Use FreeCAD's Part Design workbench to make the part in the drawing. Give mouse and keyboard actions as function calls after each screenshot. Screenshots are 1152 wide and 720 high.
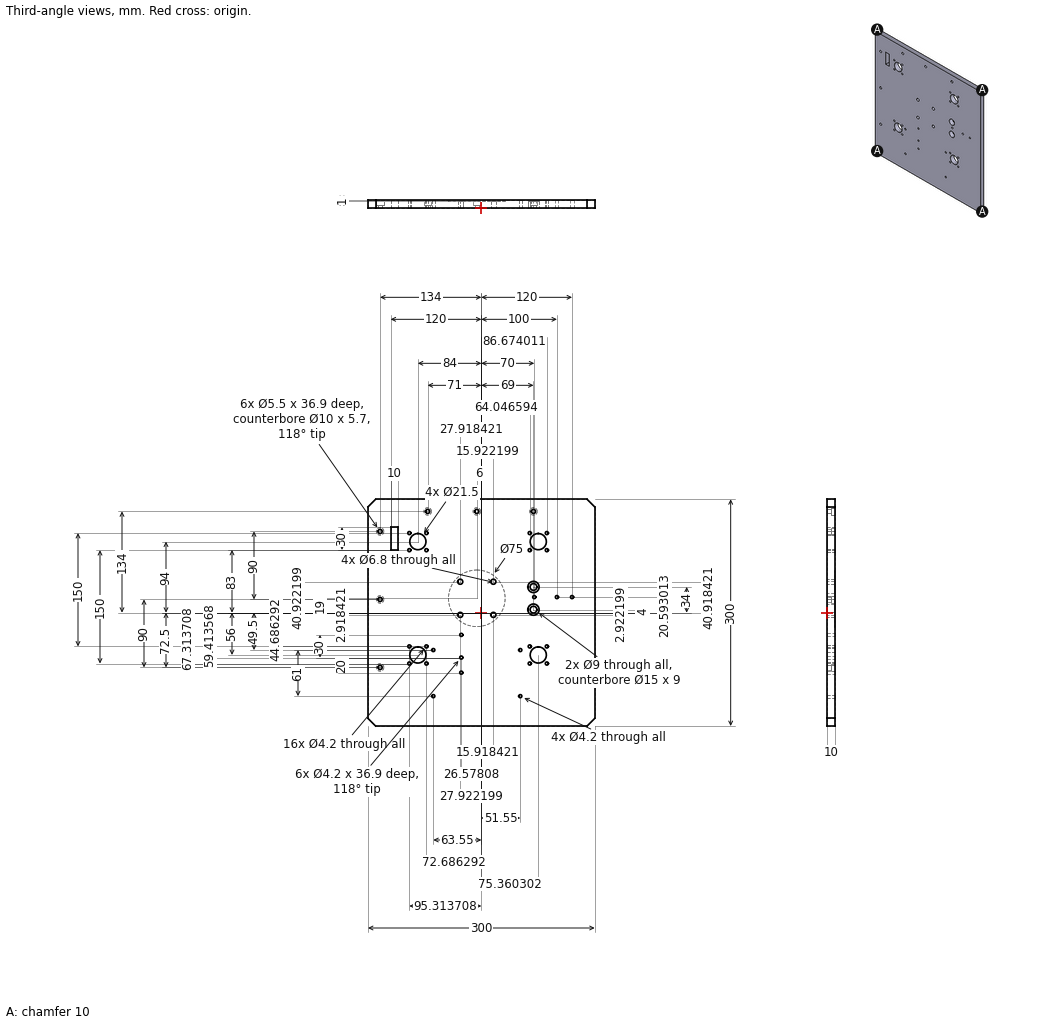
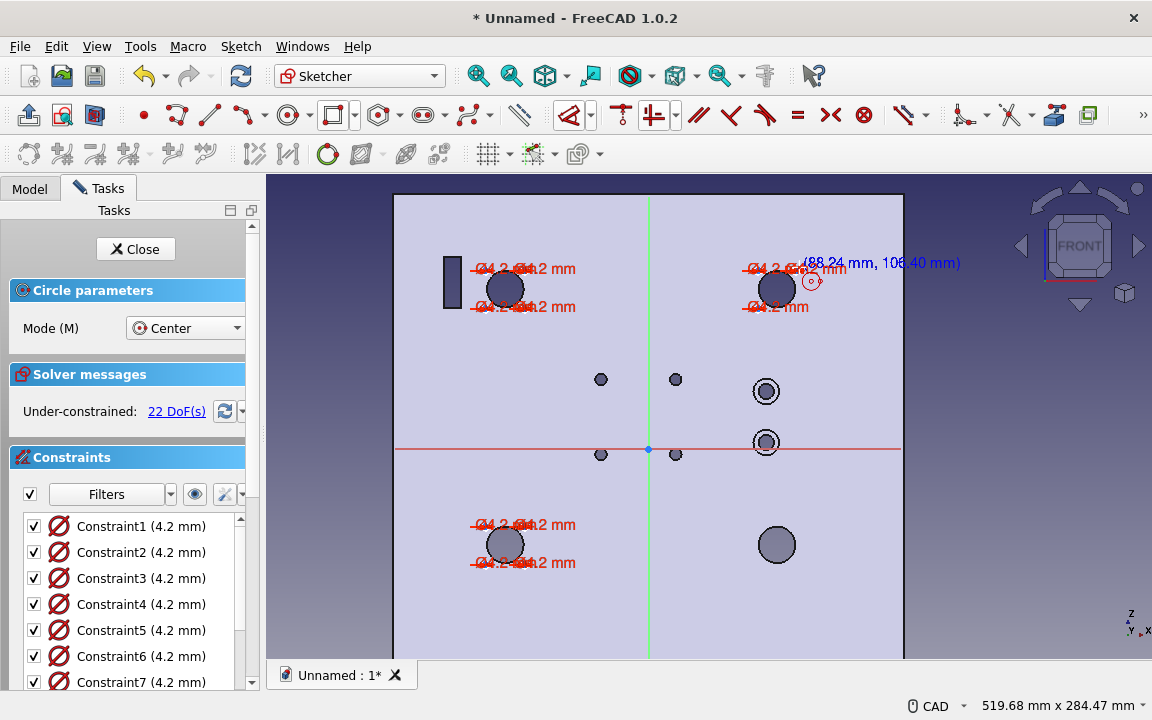
scroll(796, 308, up, 10)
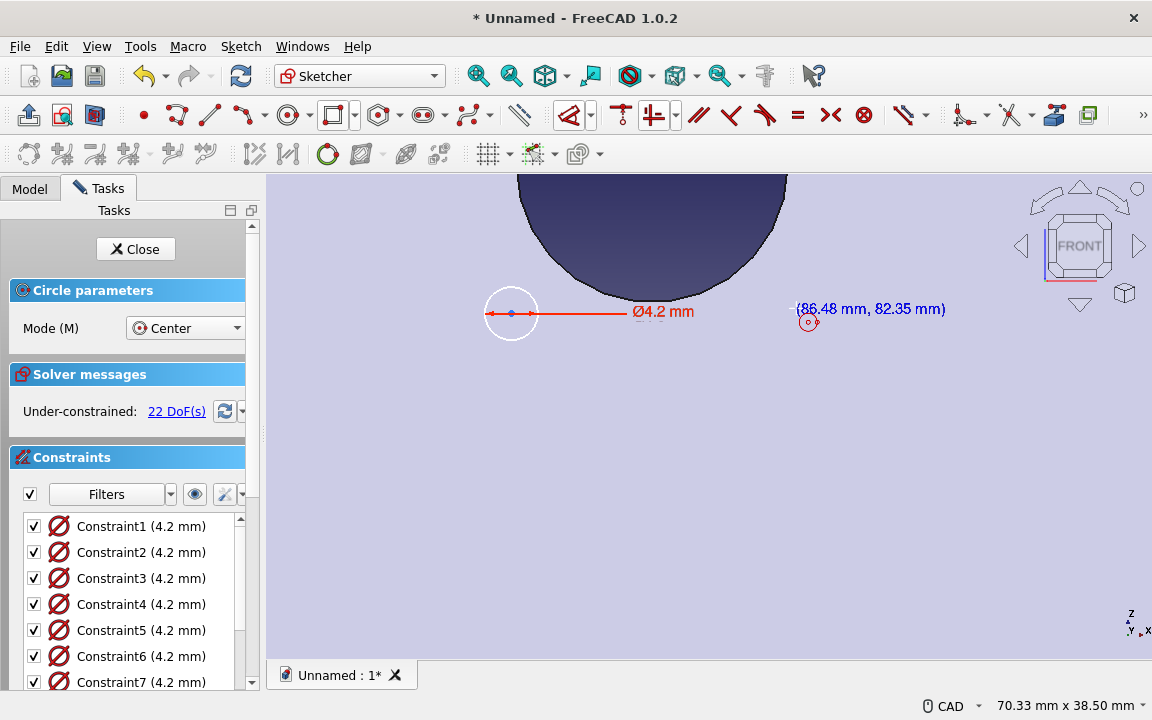
scroll(796, 308, down, 10)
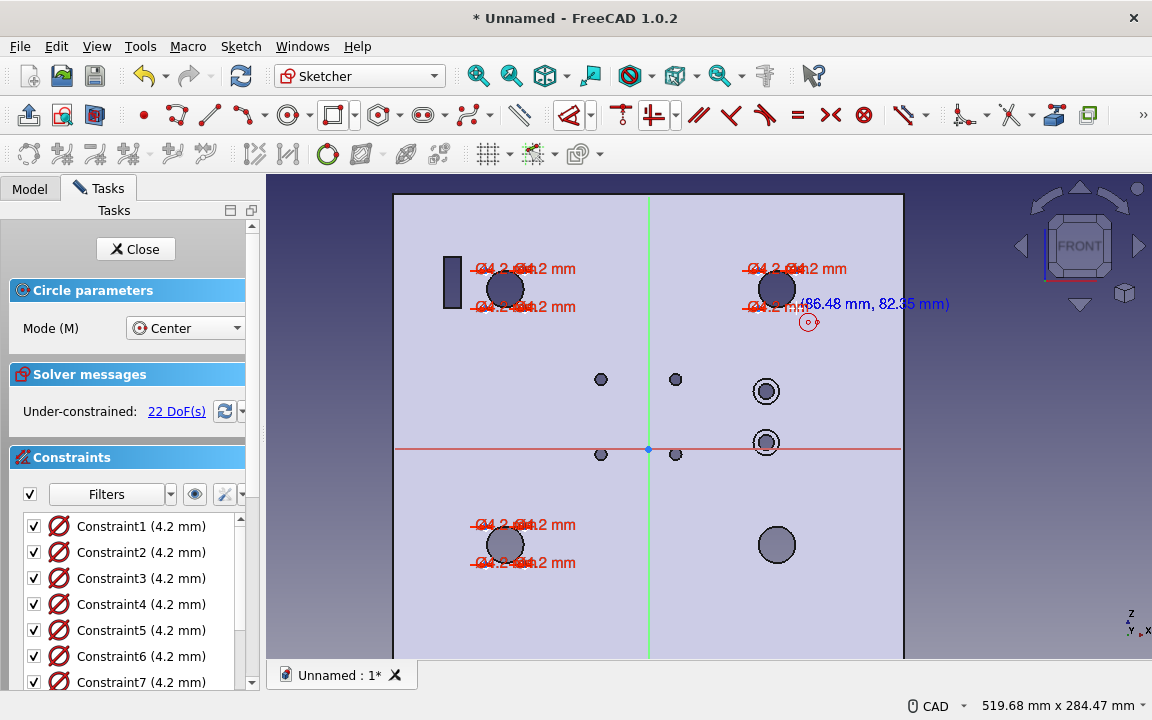
click(796, 308)
move(799, 306)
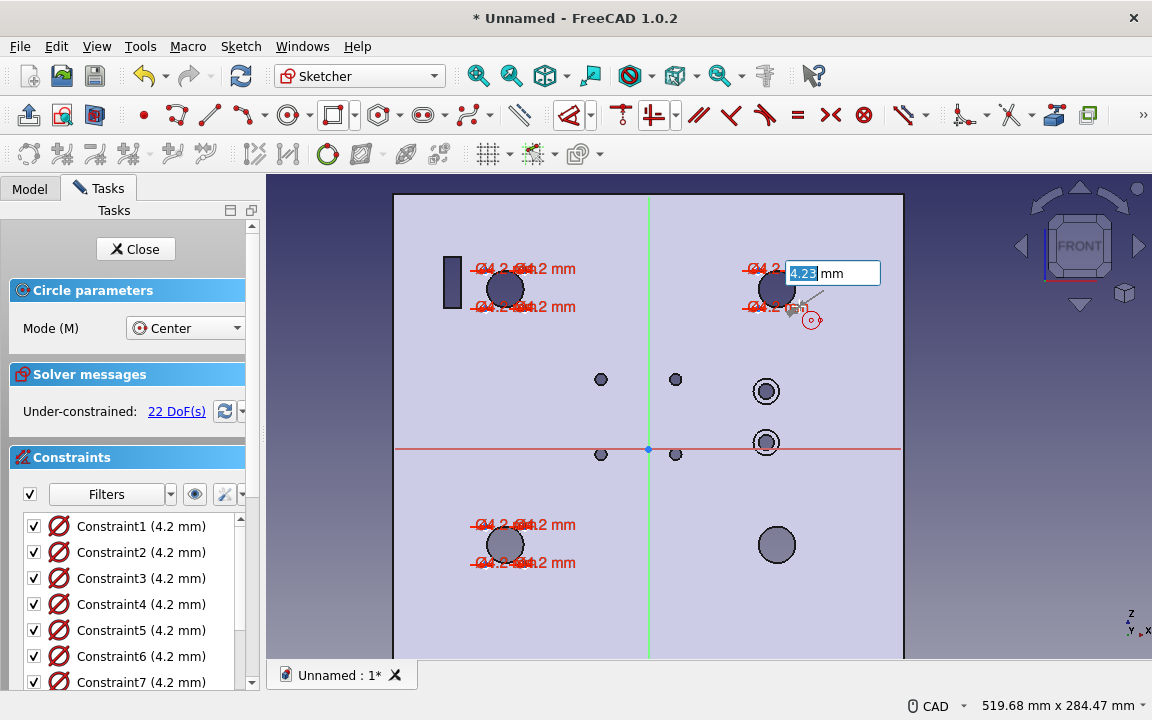
text(4.2)
key(Return)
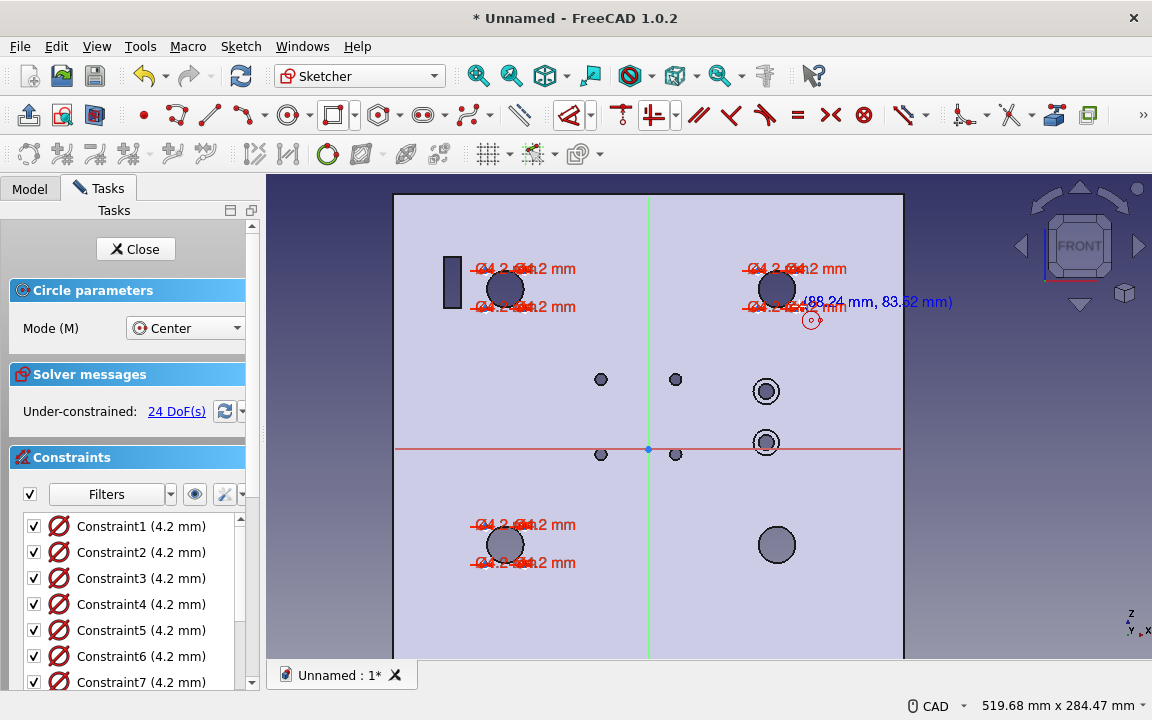
scroll(758, 564, up, 10)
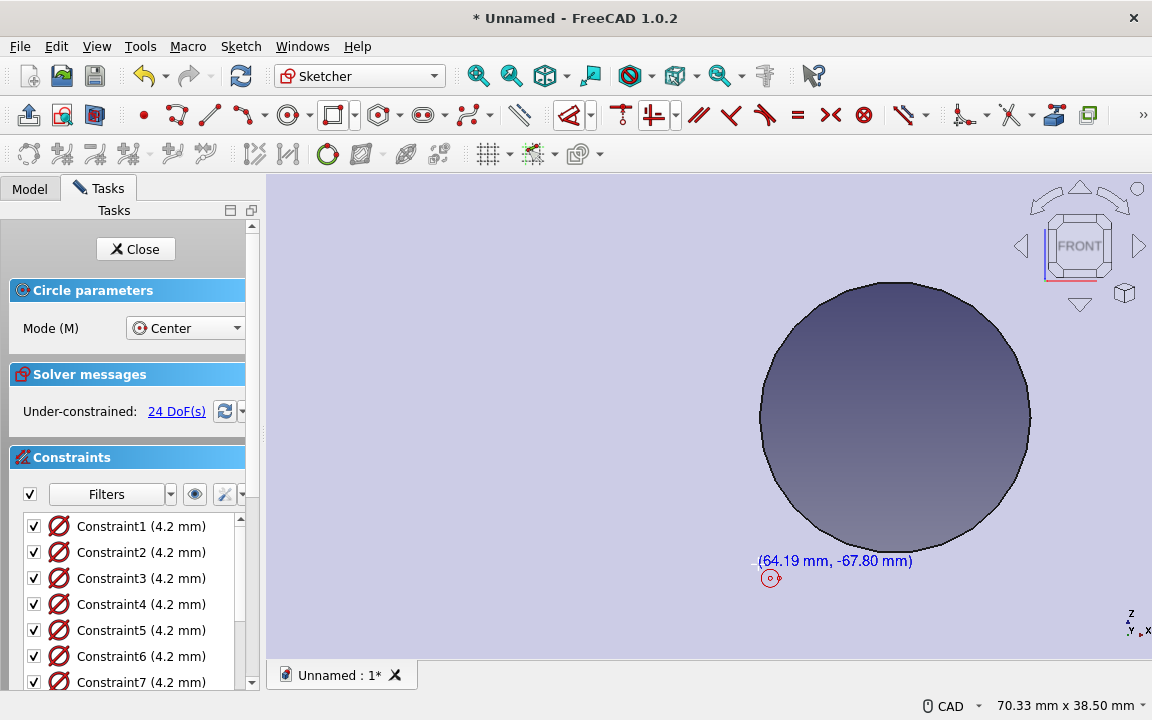
scroll(758, 564, down, 10)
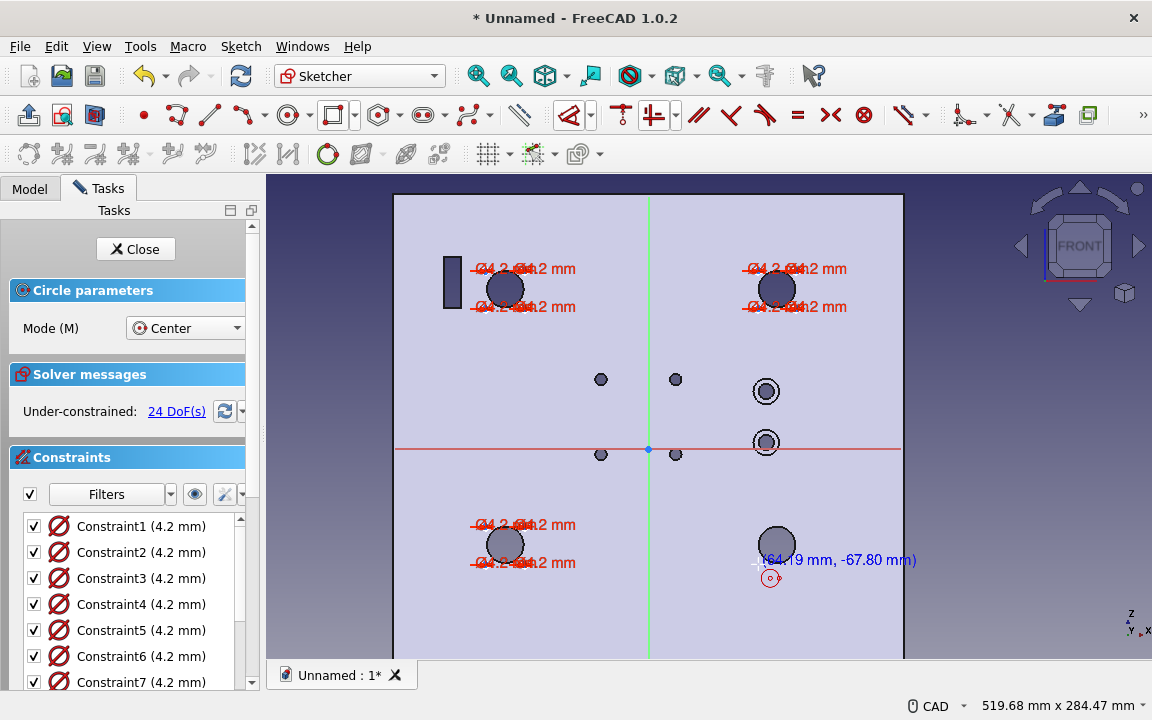
click(758, 564)
move(760, 562)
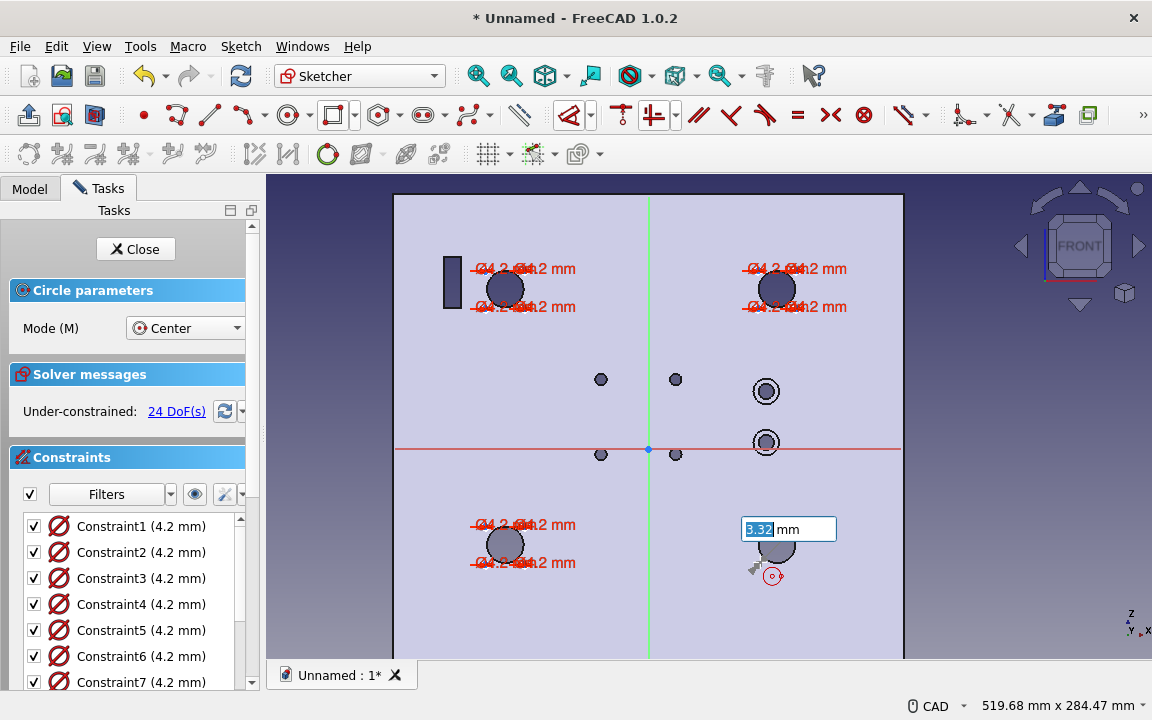
text(4.2)
key(Return)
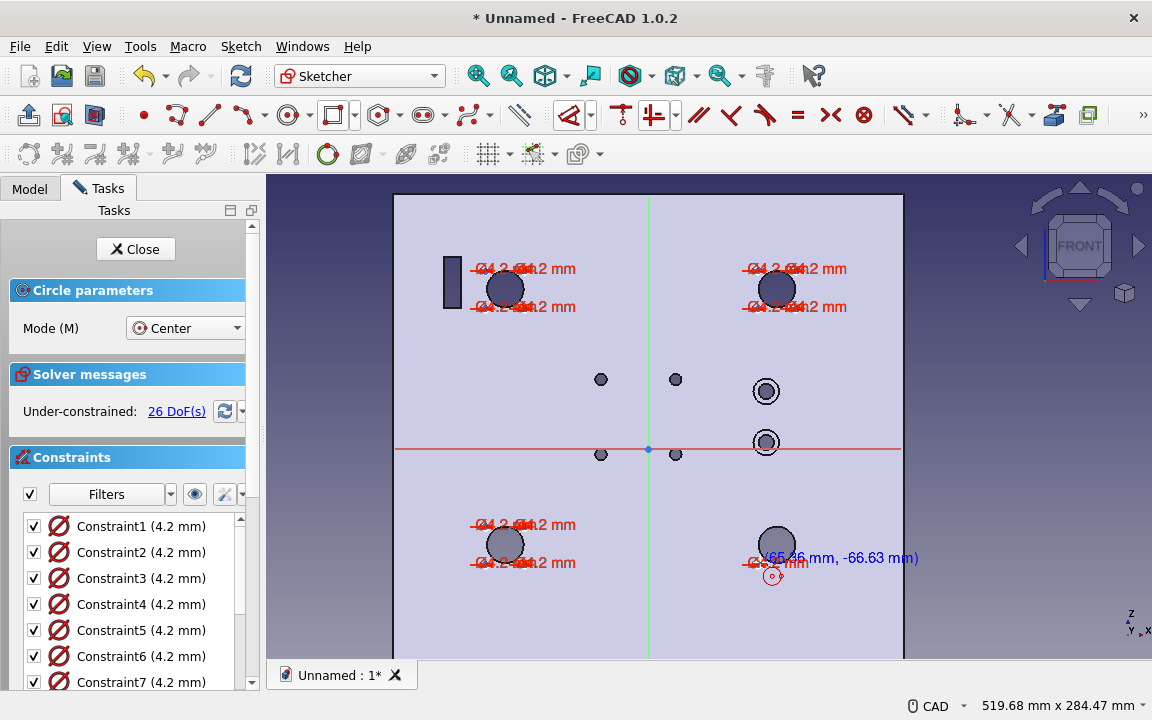
scroll(758, 526, up, 10)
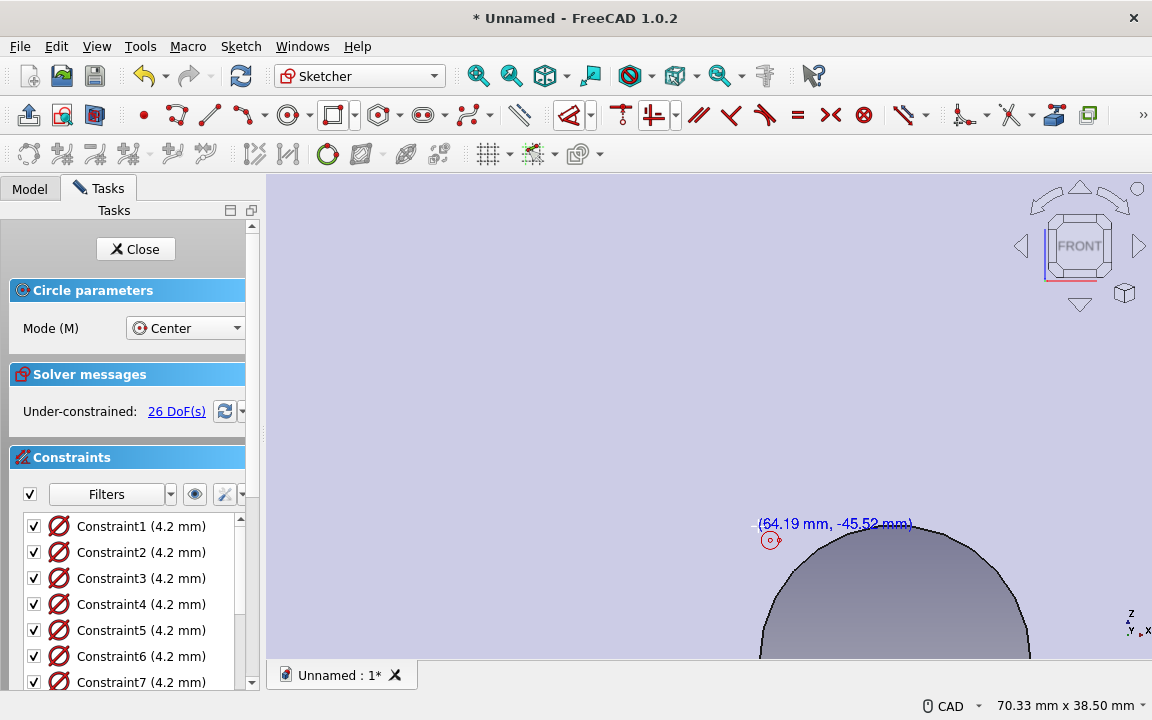
scroll(758, 526, down, 10)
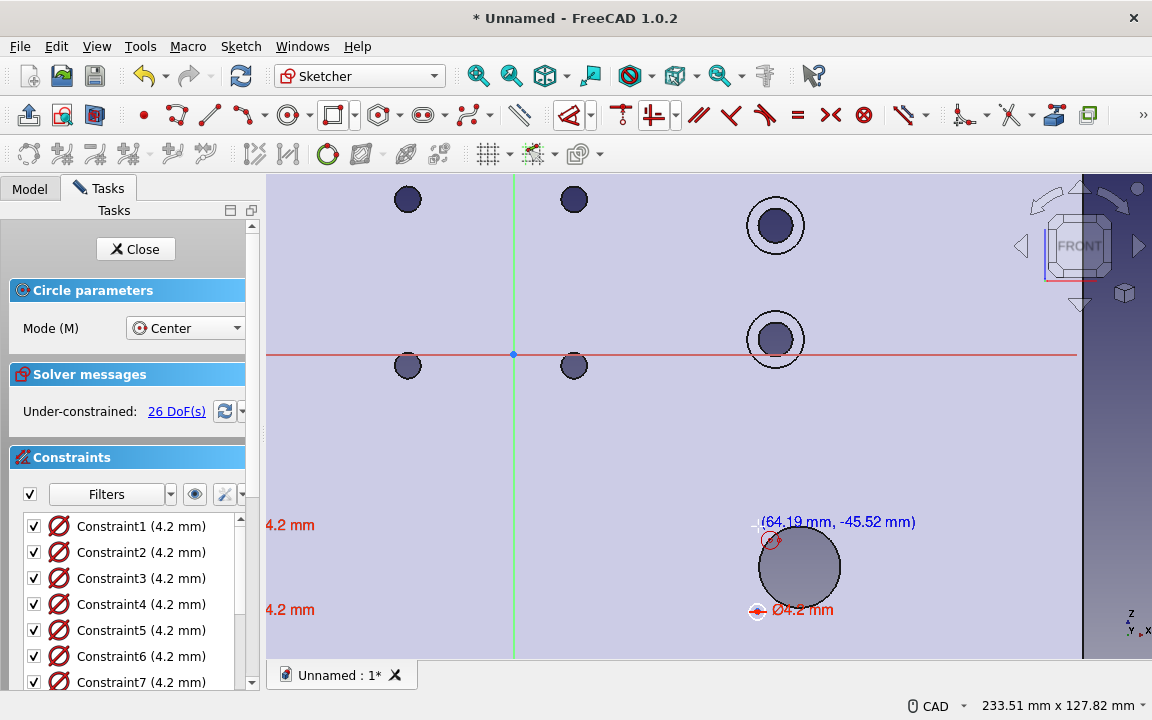
click(758, 526)
move(760, 523)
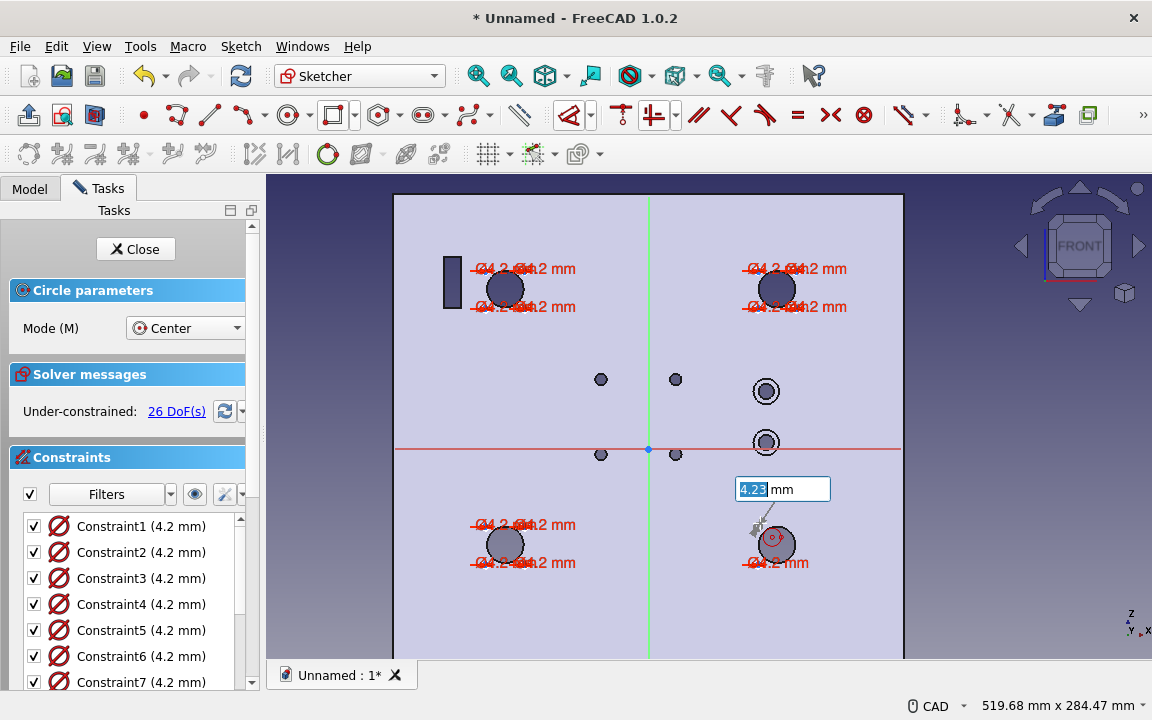
text(4.2)
key(Return)